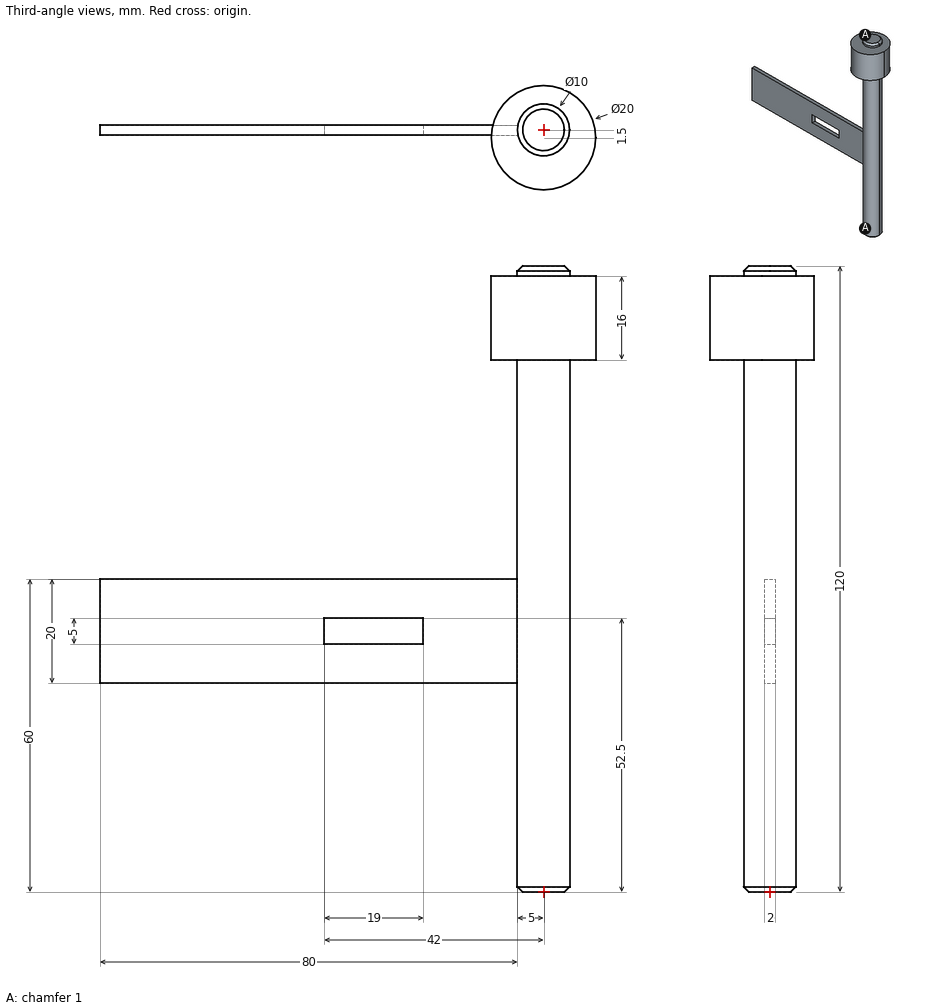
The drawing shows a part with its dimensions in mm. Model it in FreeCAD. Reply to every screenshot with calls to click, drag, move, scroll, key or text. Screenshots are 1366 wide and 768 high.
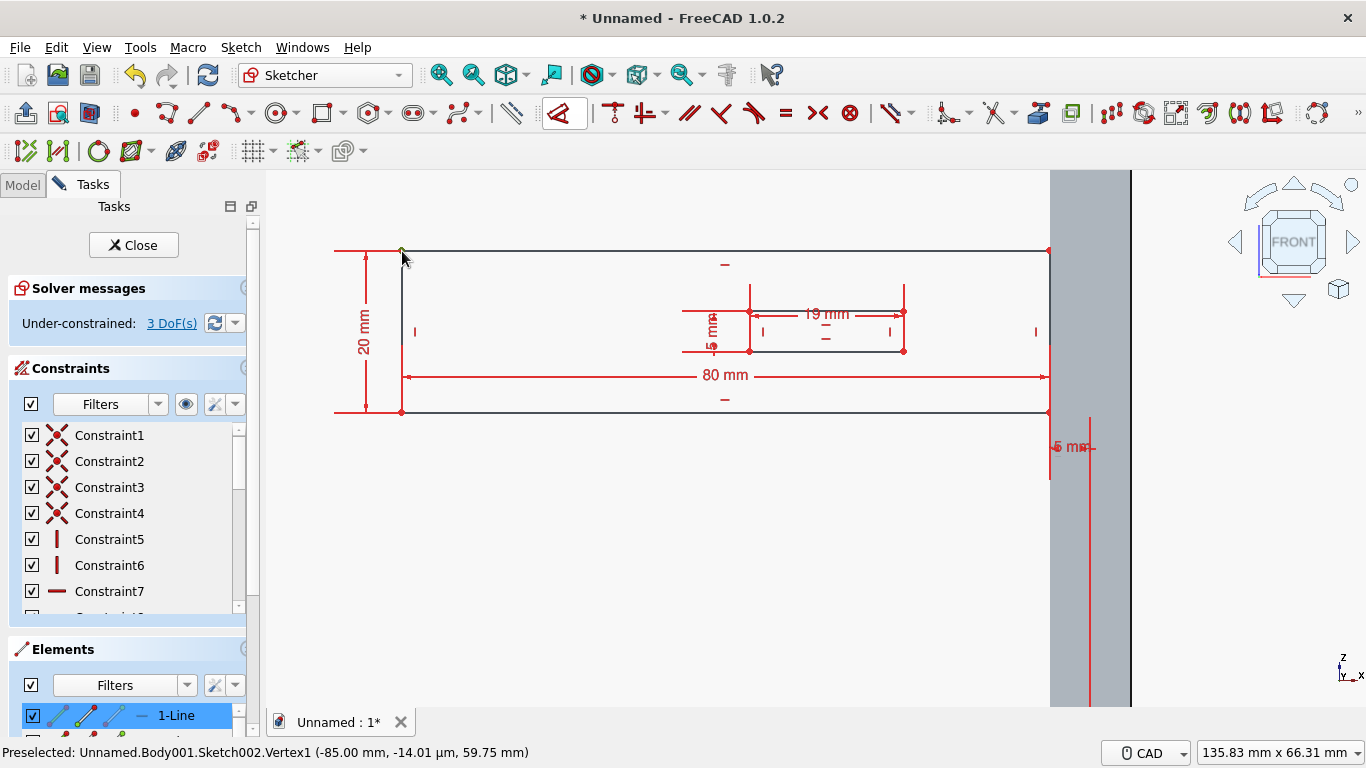
key(i)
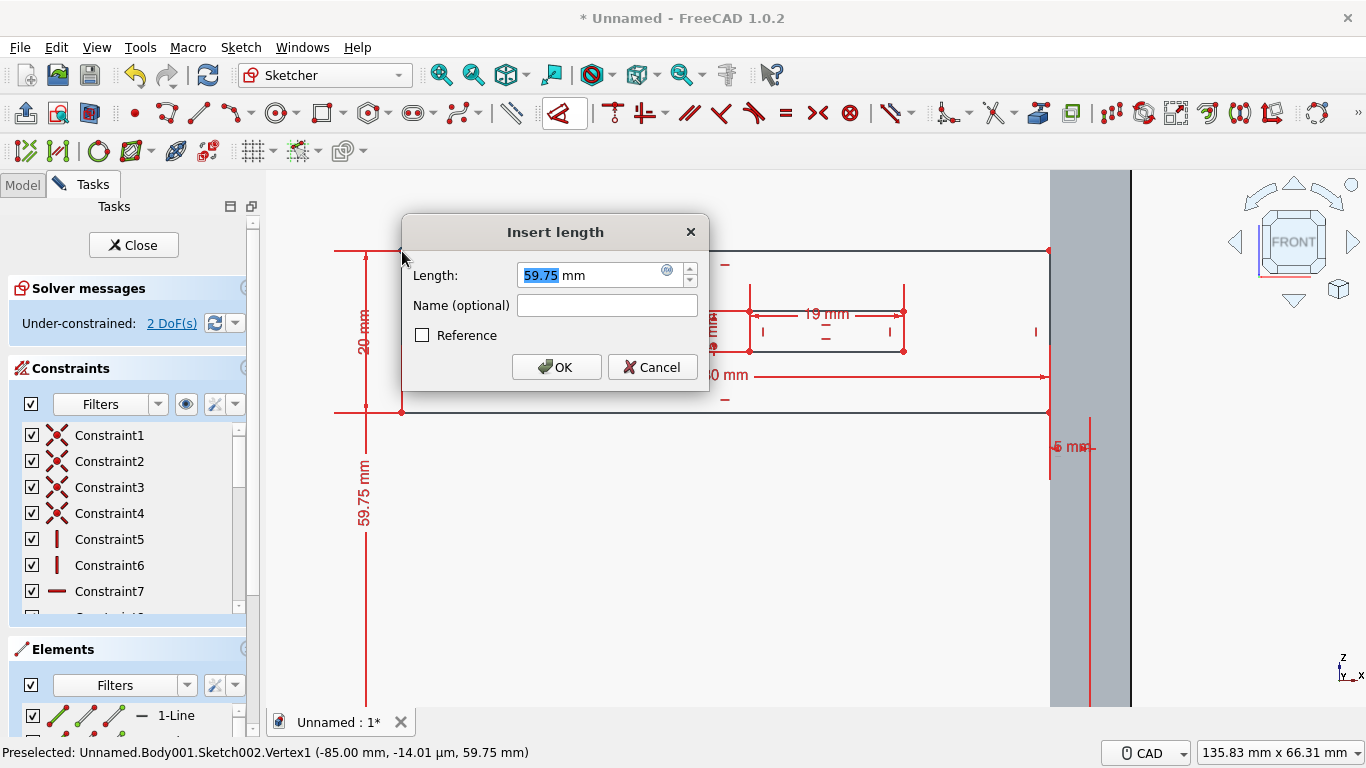
text(60)
key(Return)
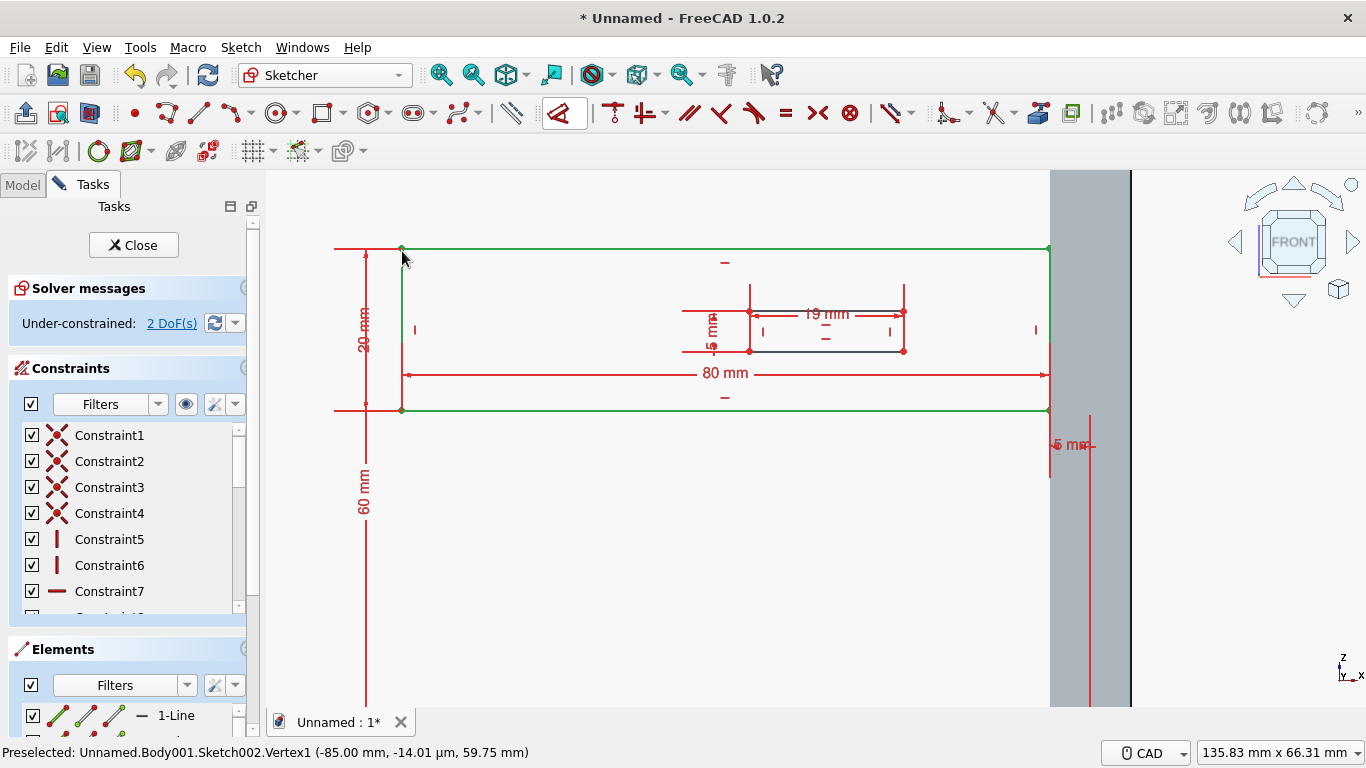
click(750, 311)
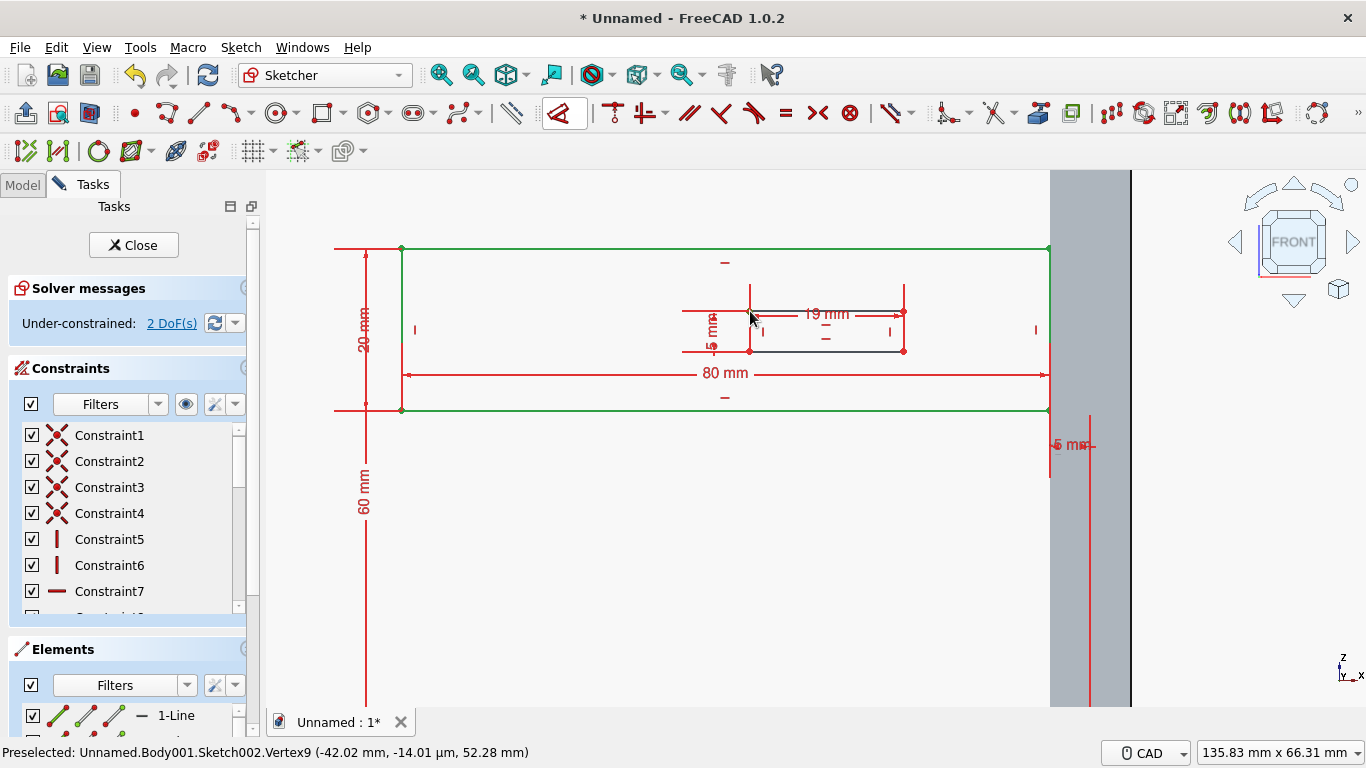
click(582, 114)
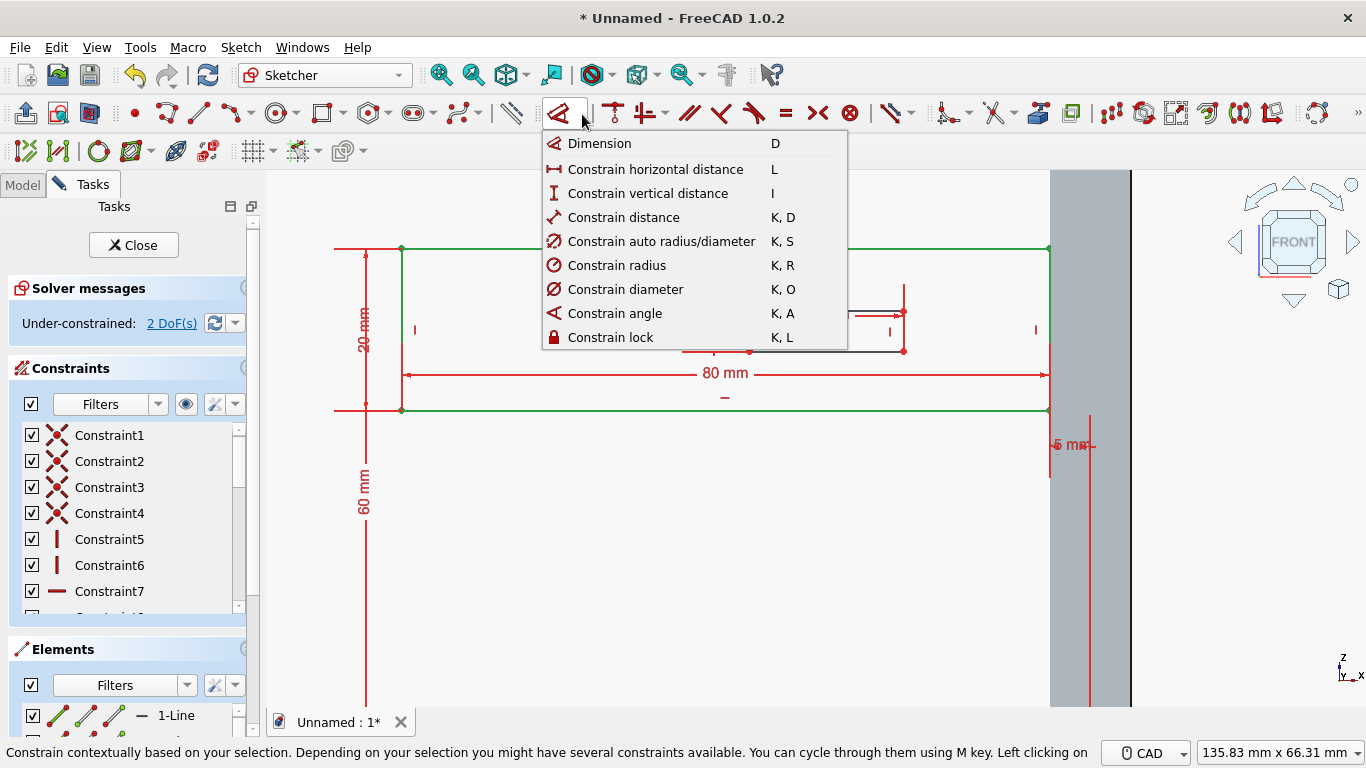
click(695, 169)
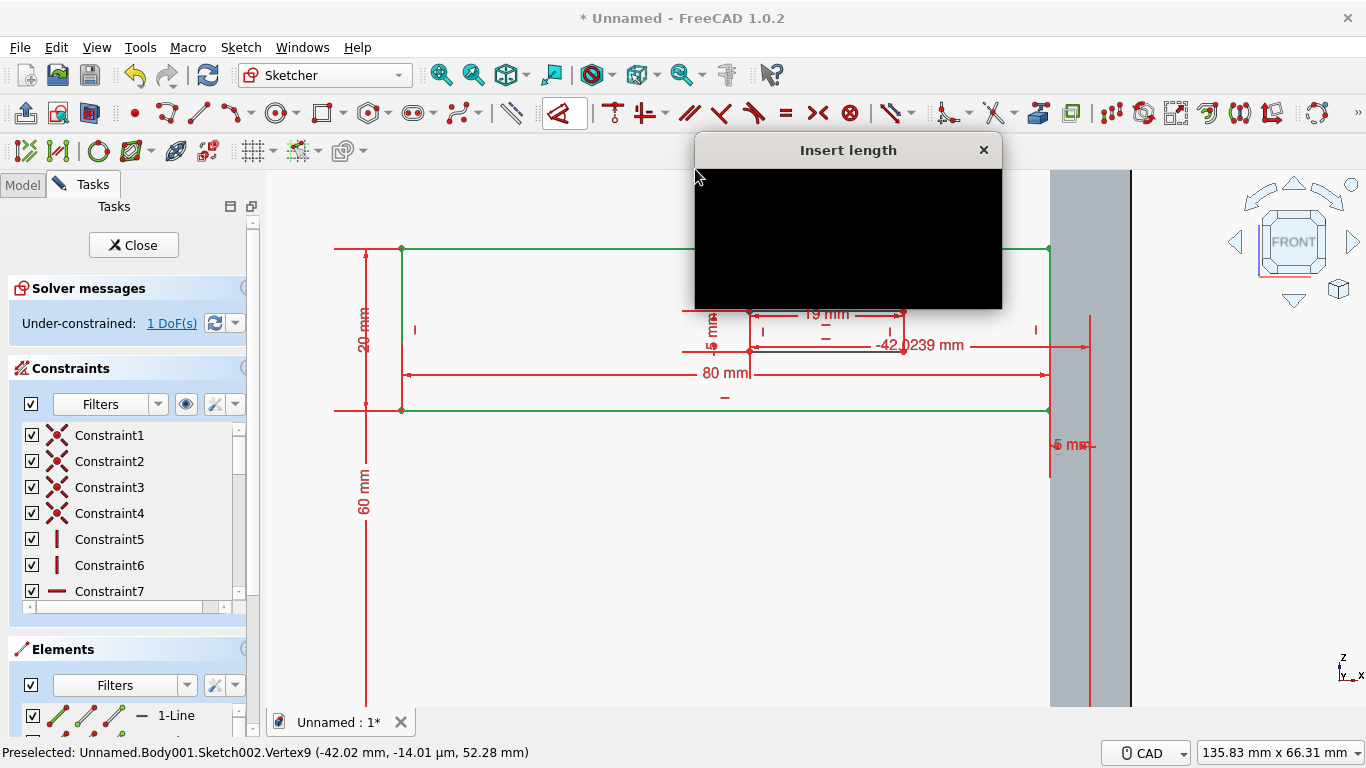
text(-42)
key(Return)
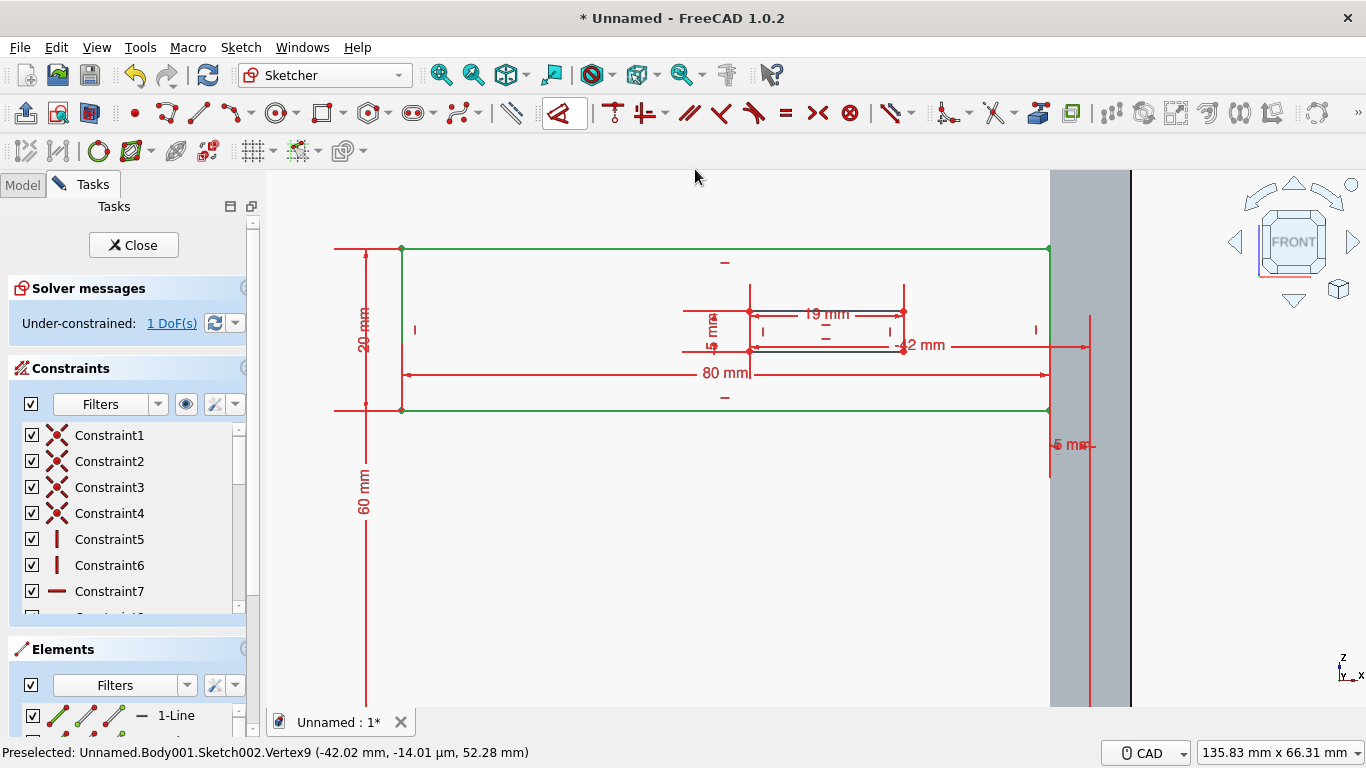
click(750, 311)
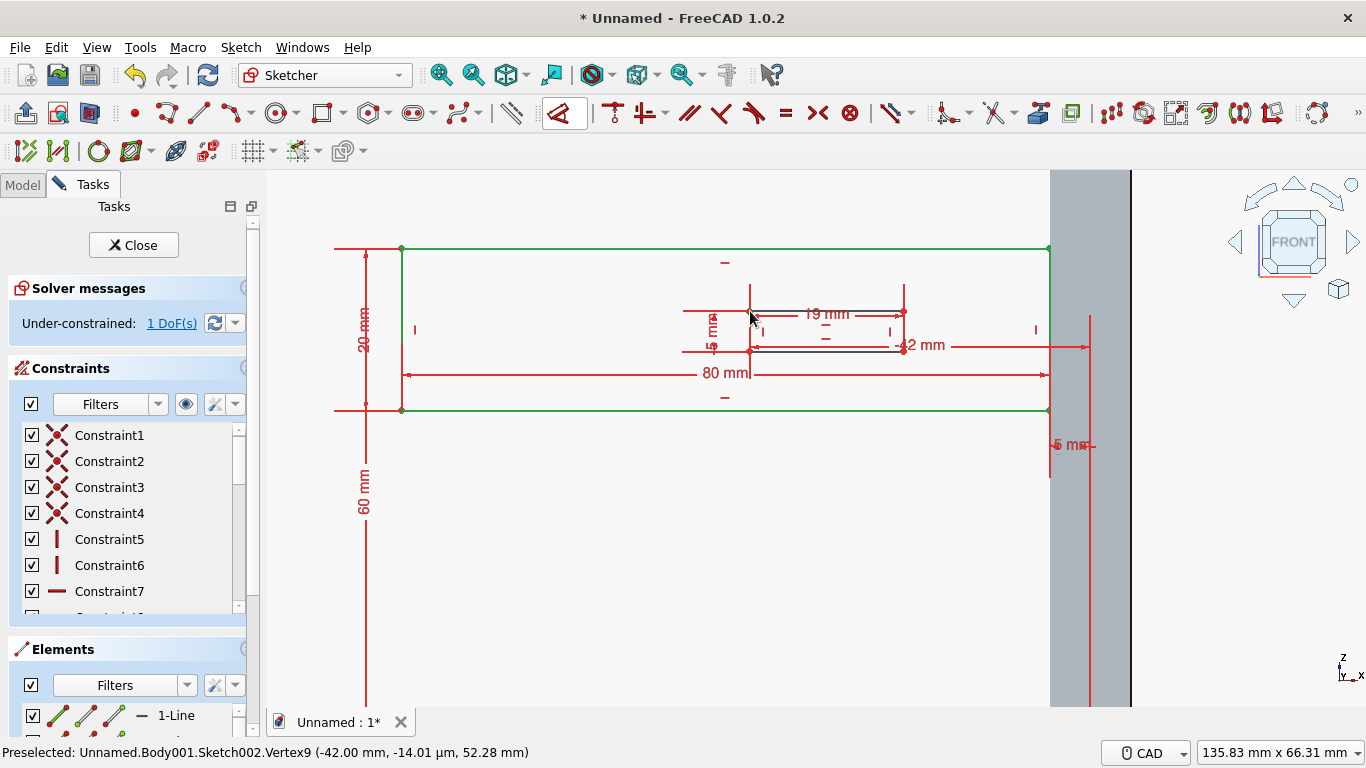
key(i)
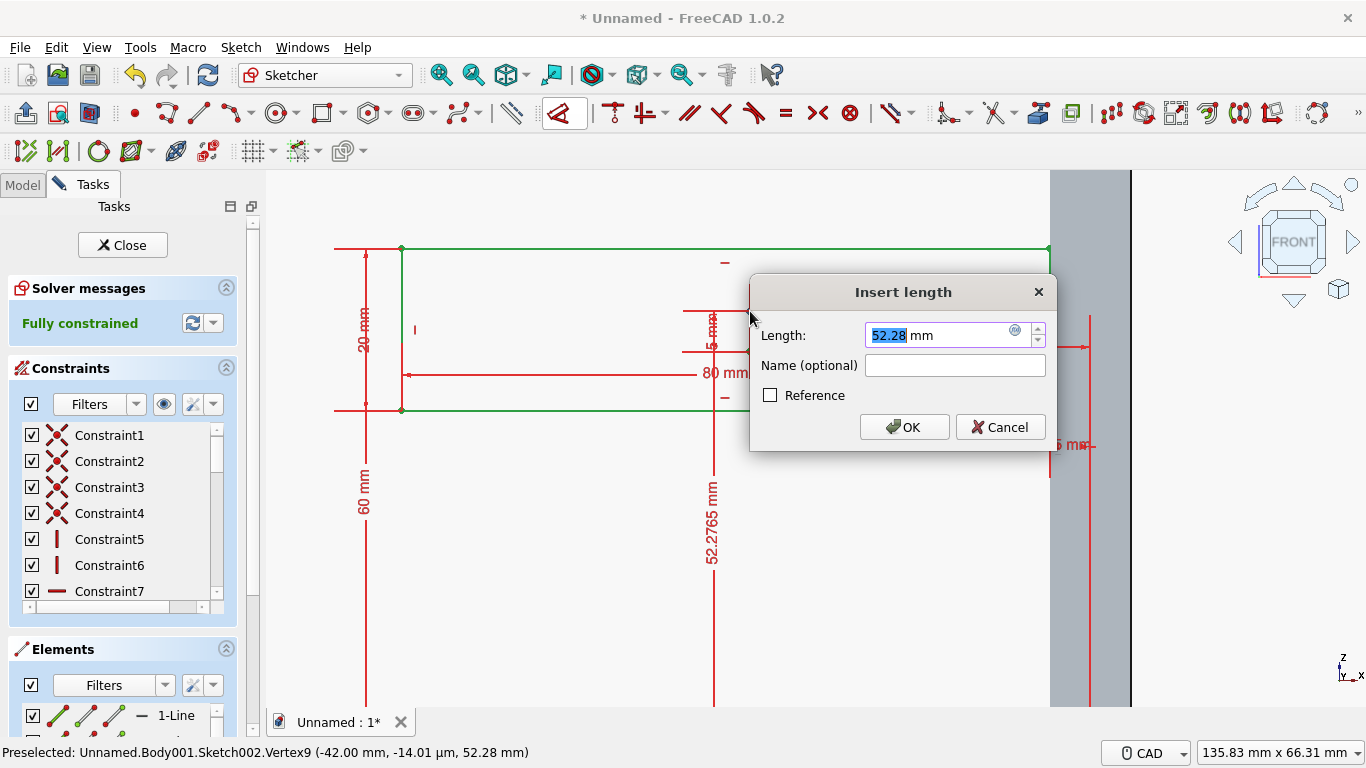
text(52.5)
key(Return)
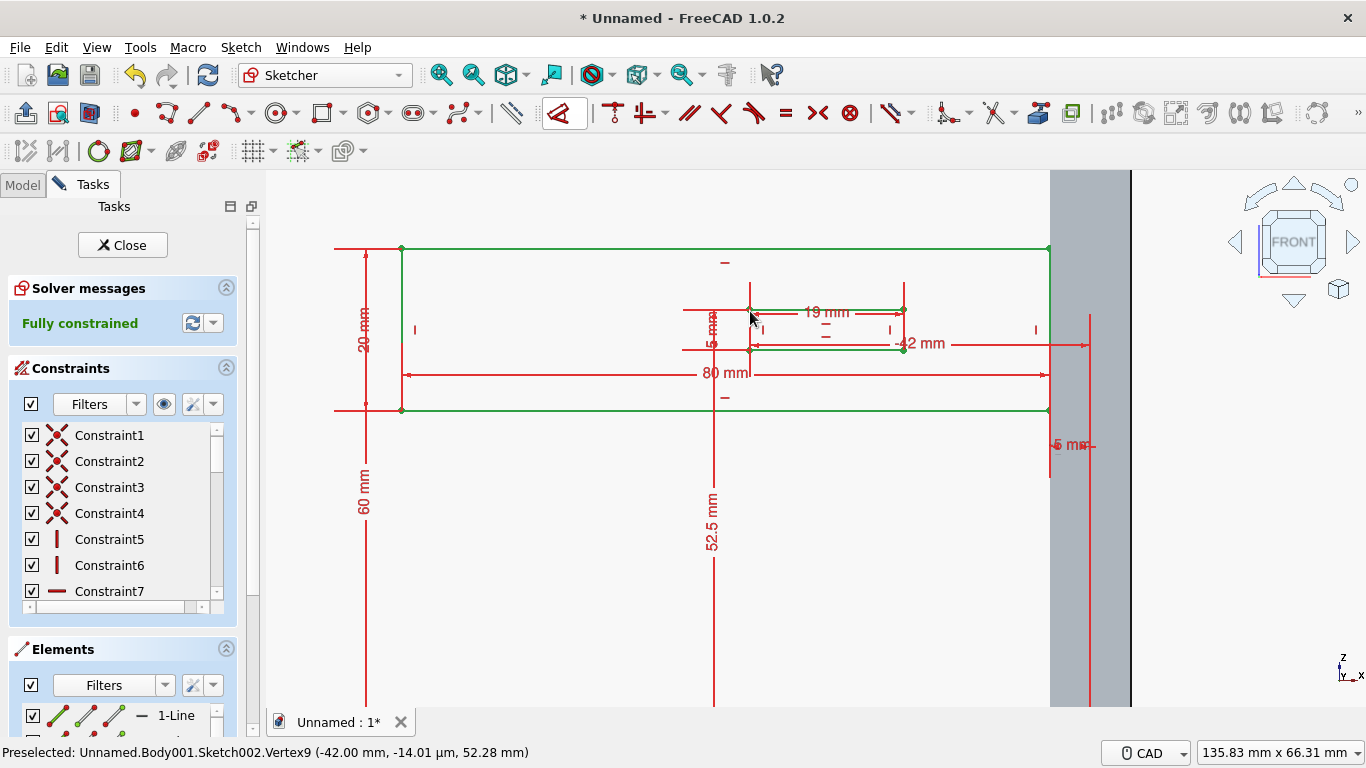
click(123, 245)